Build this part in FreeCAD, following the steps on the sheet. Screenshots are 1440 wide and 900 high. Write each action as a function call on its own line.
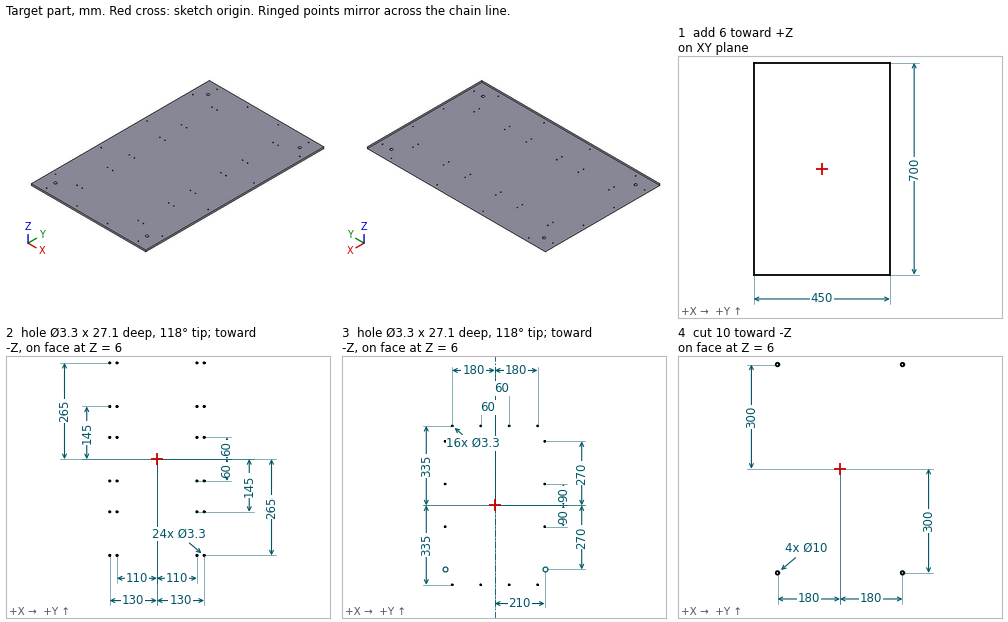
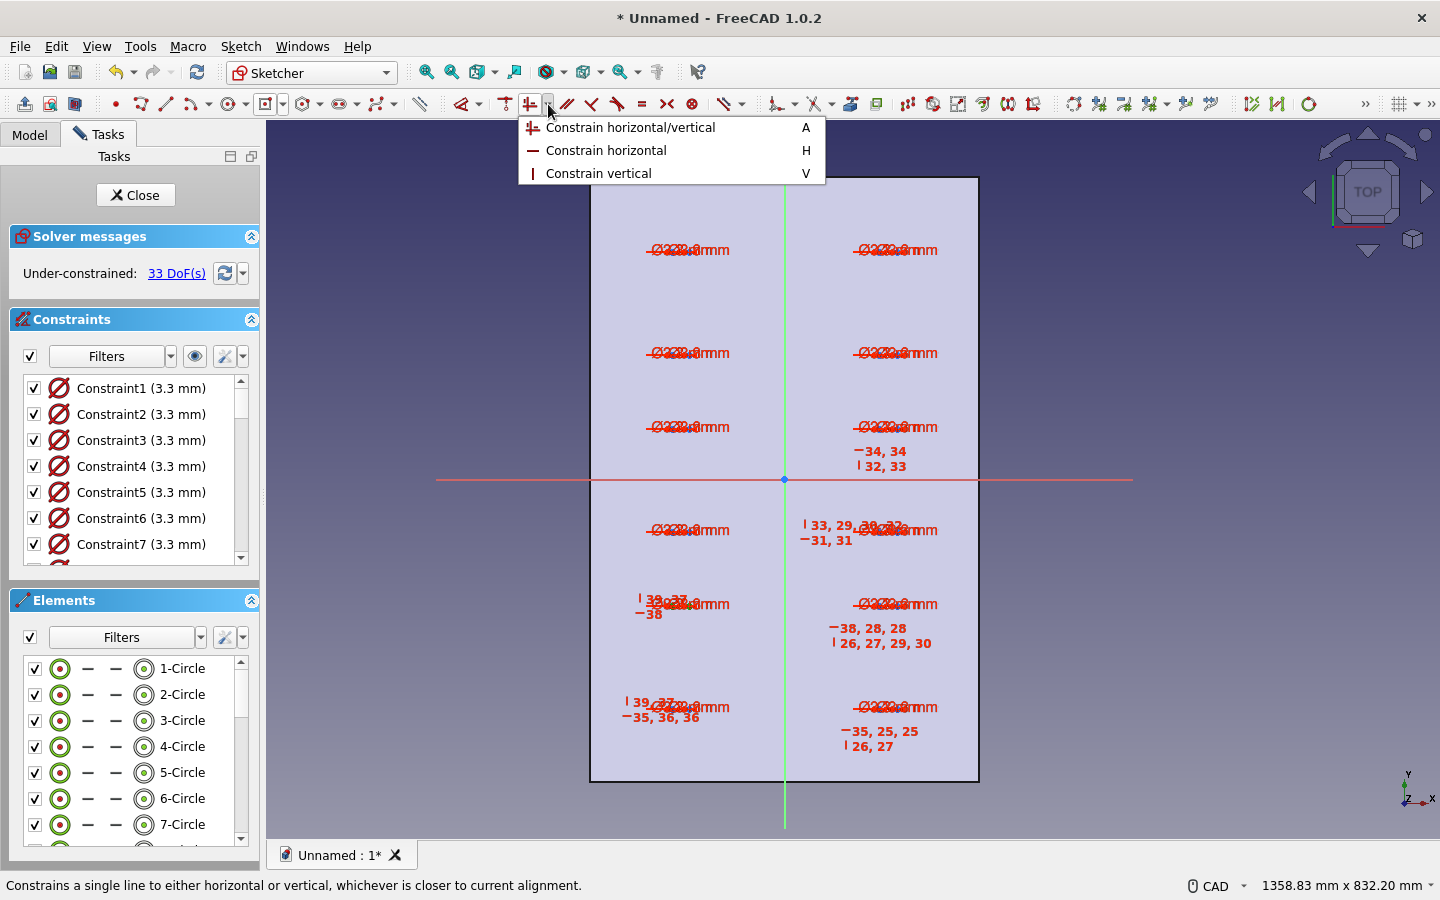
click(672, 150)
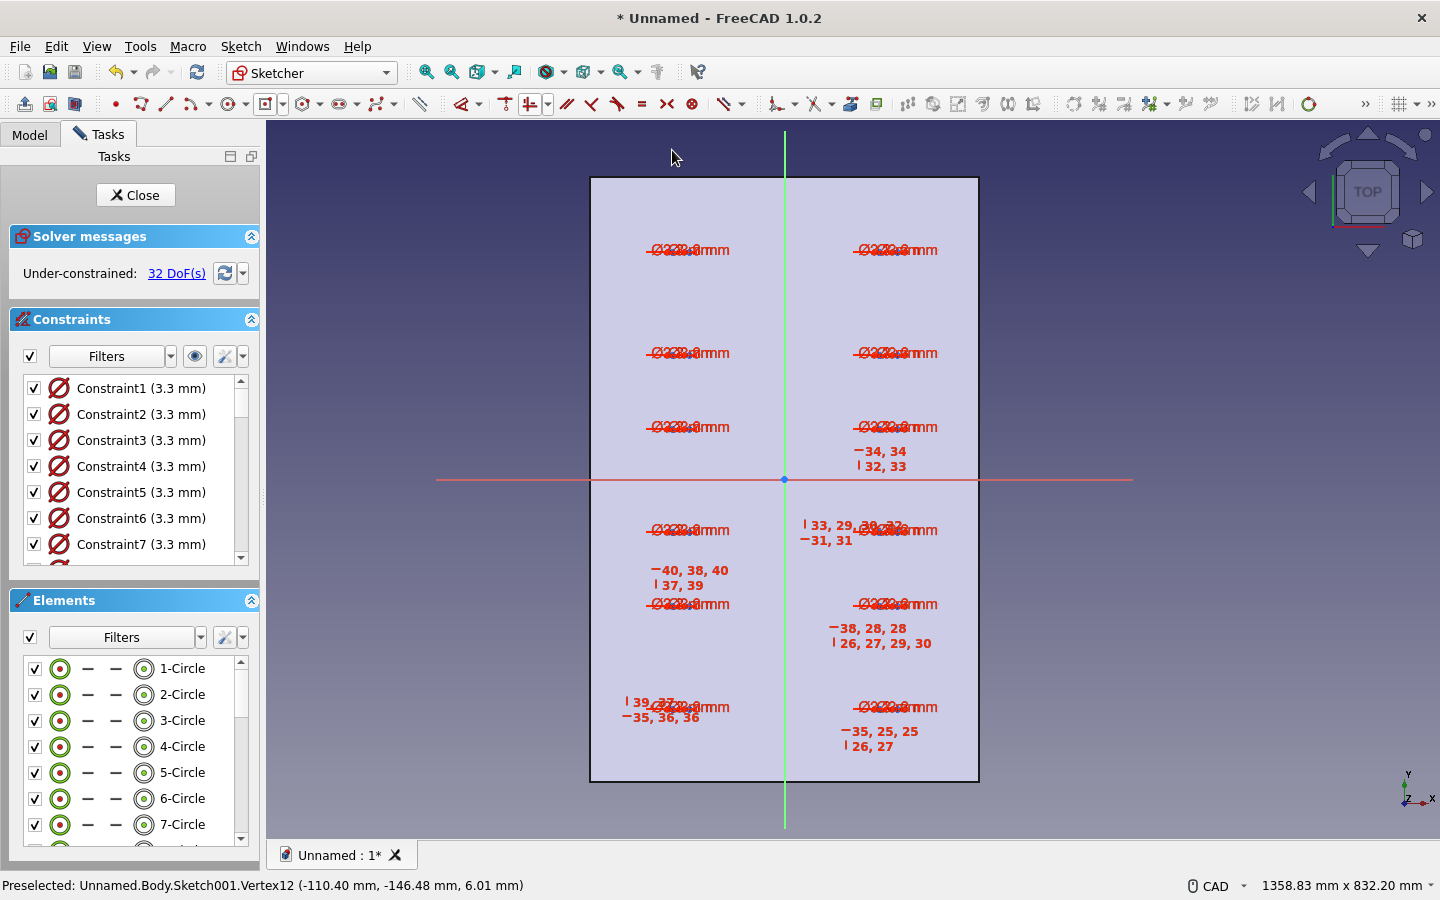
click(672, 606)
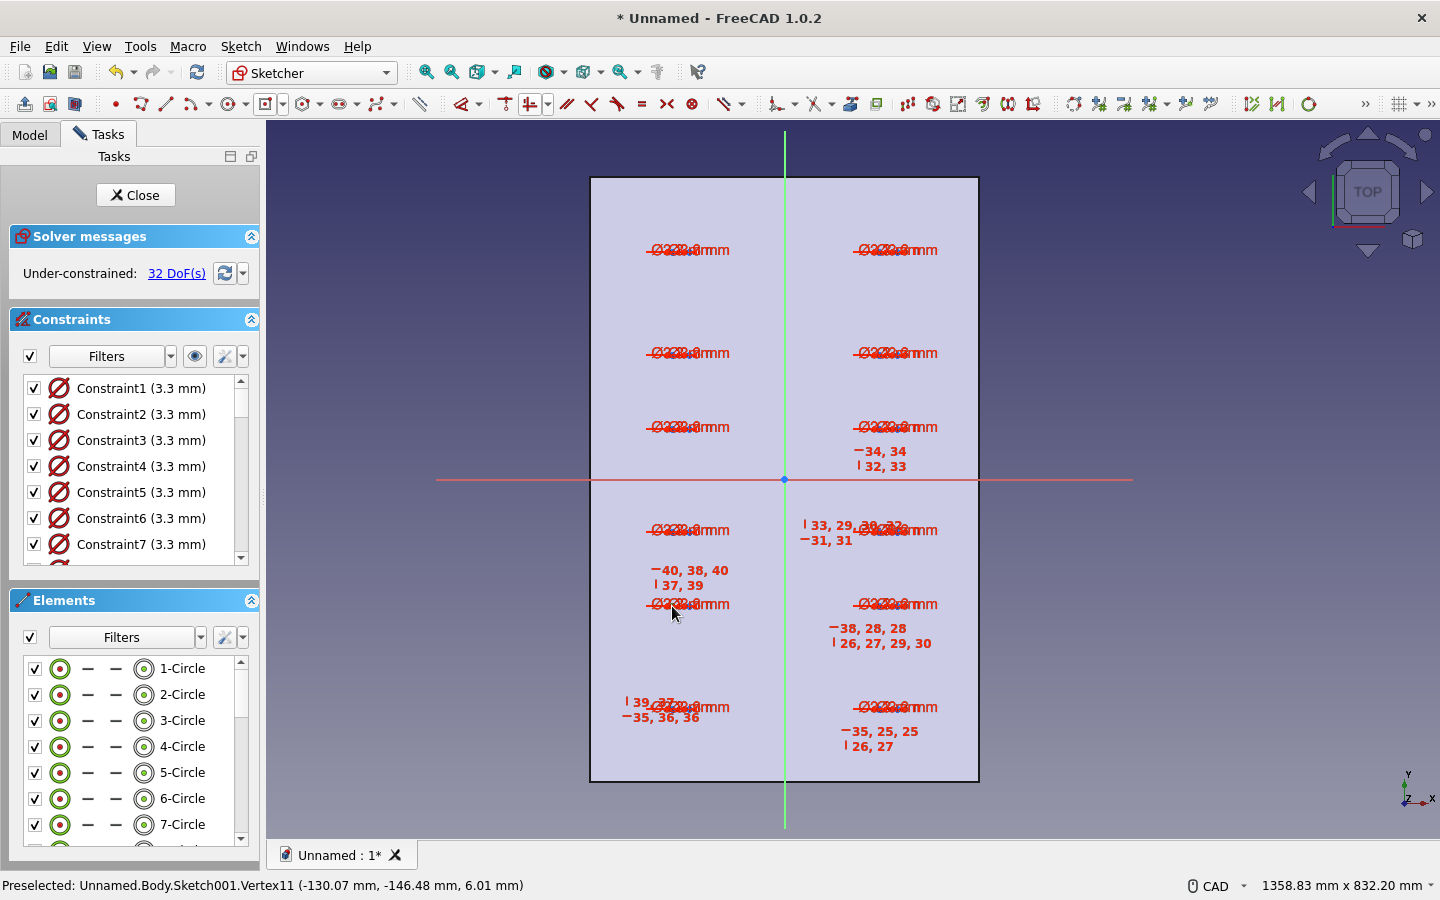
click(672, 532)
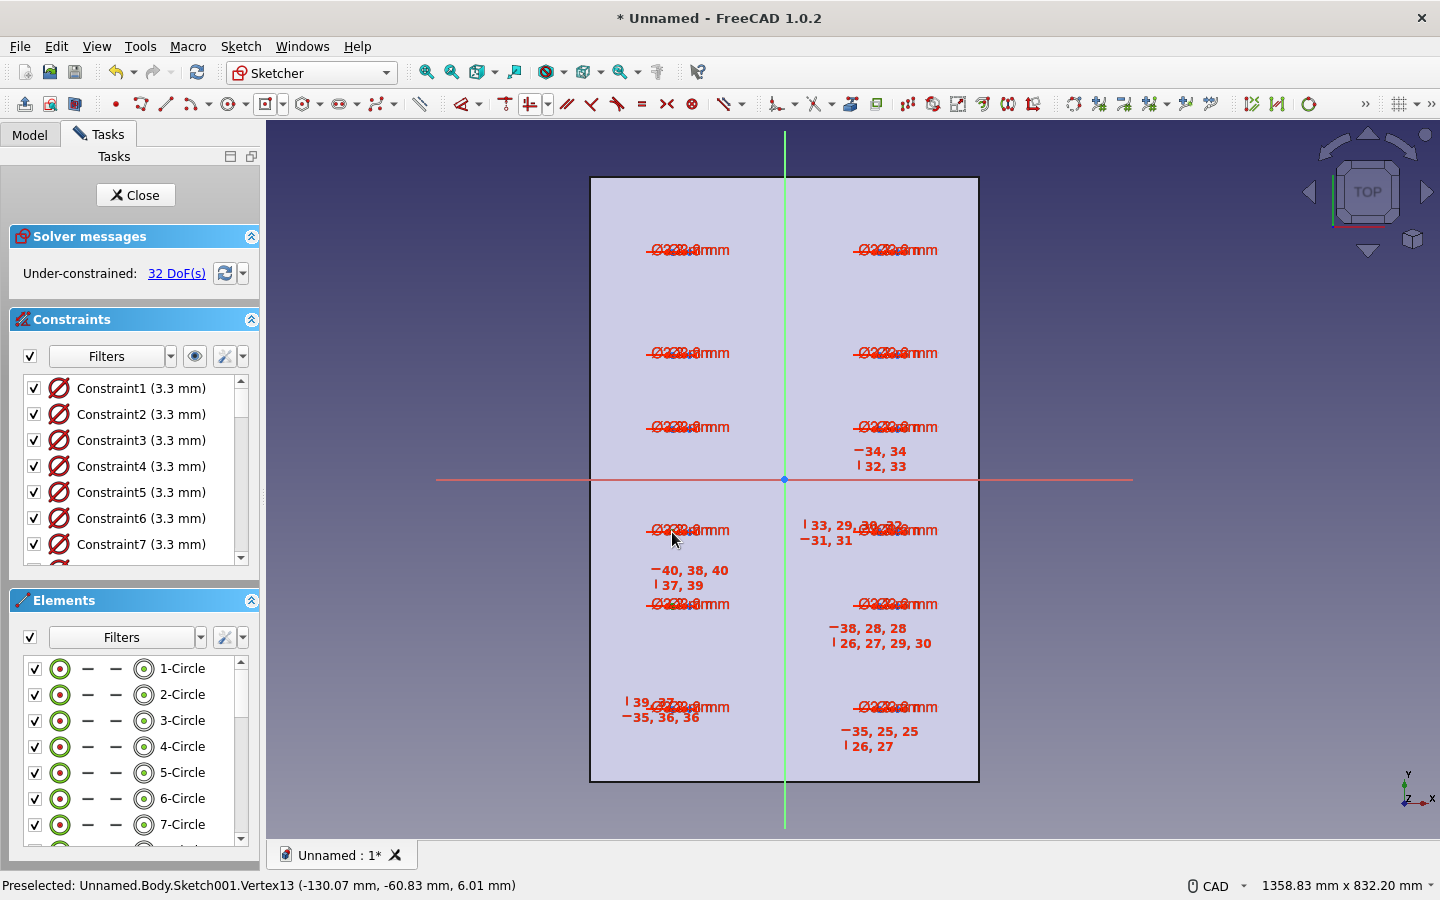
key(v)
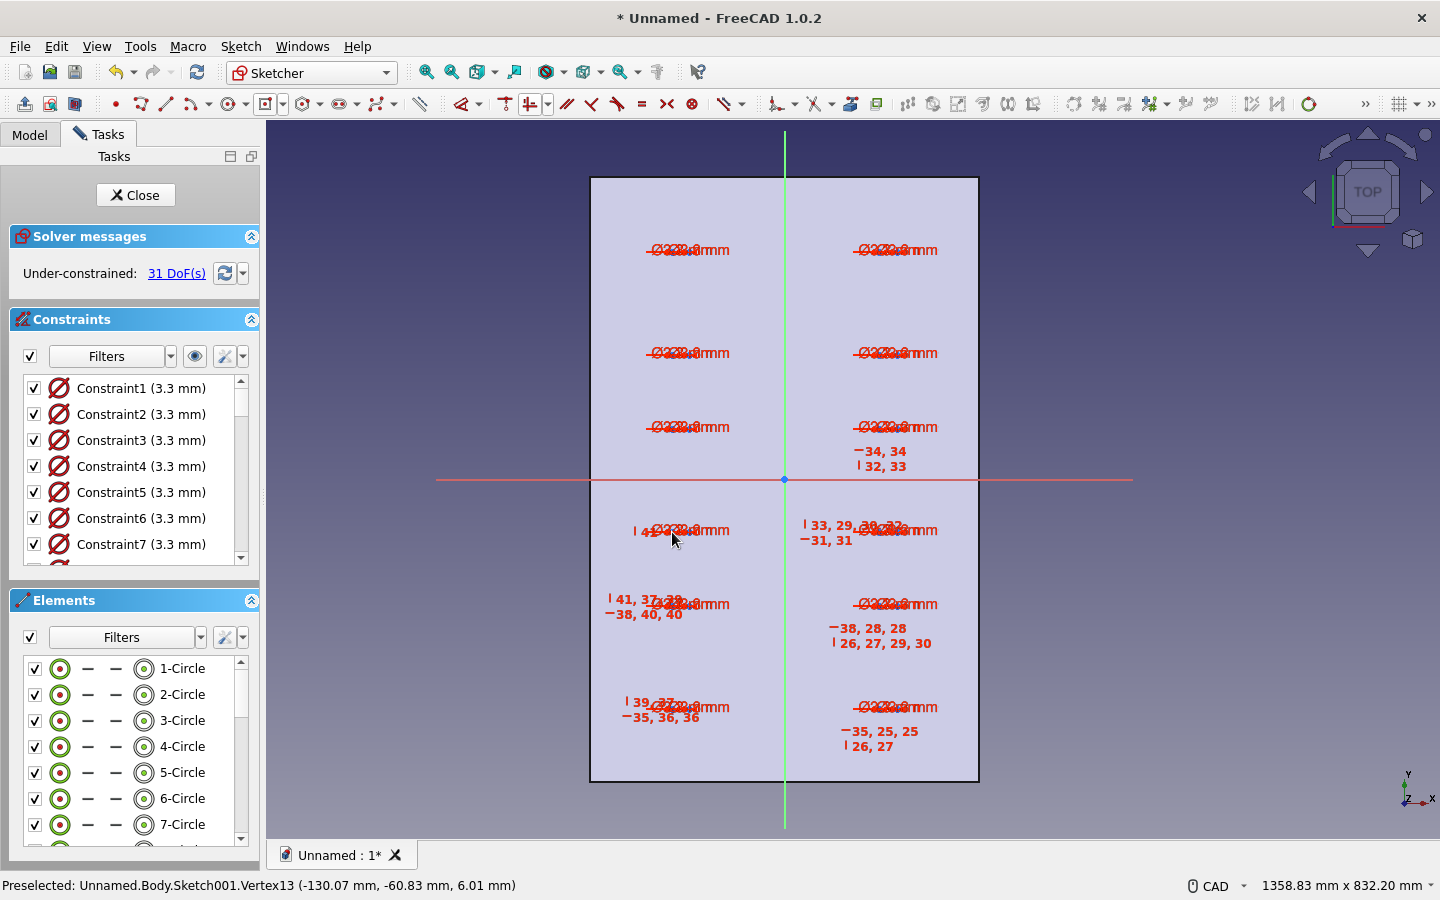
click(879, 532)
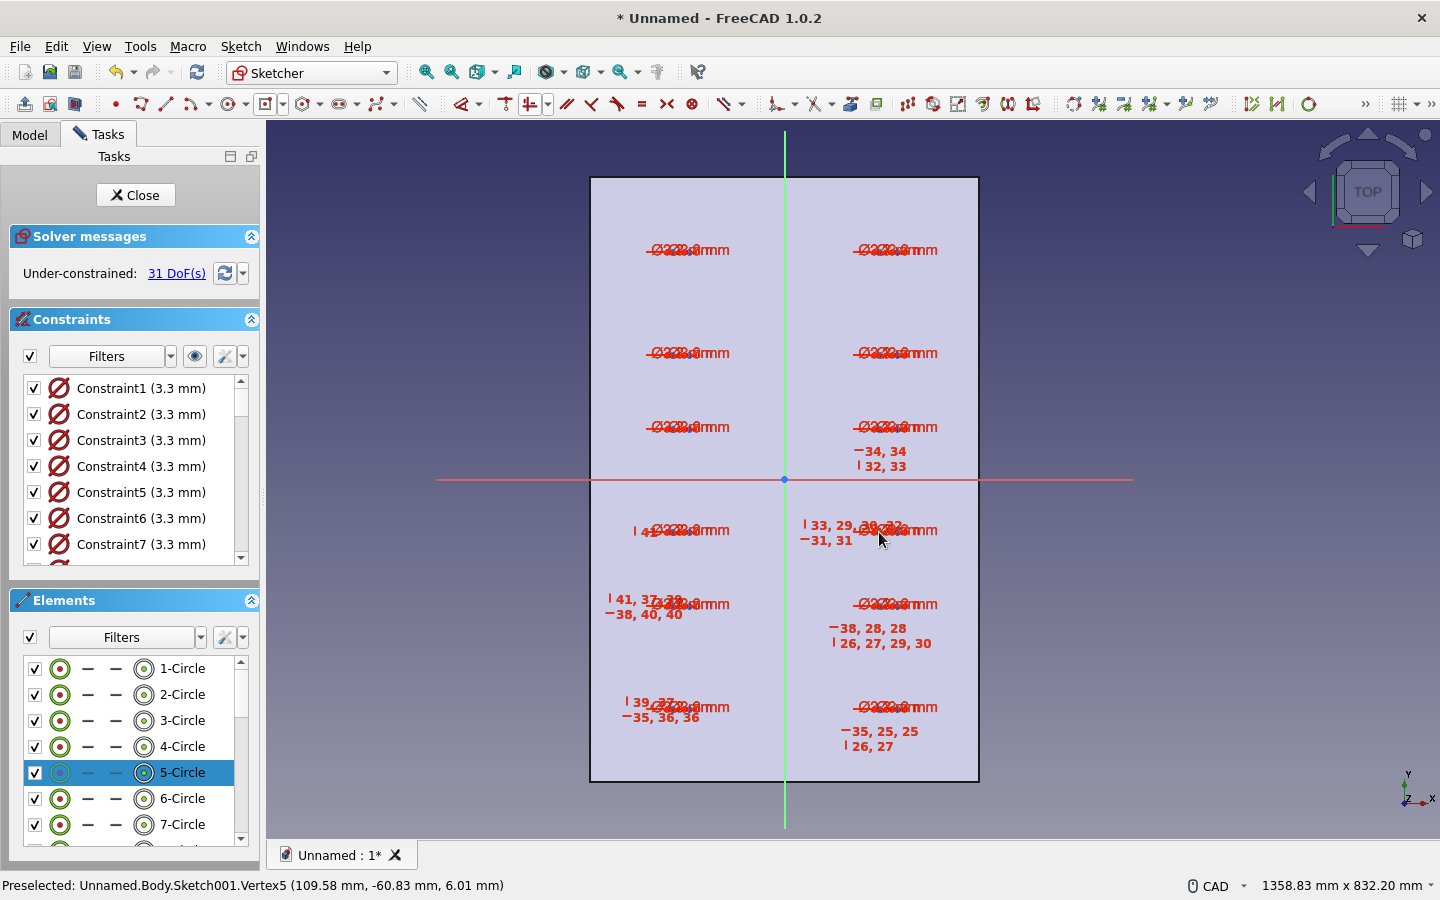
click(672, 532)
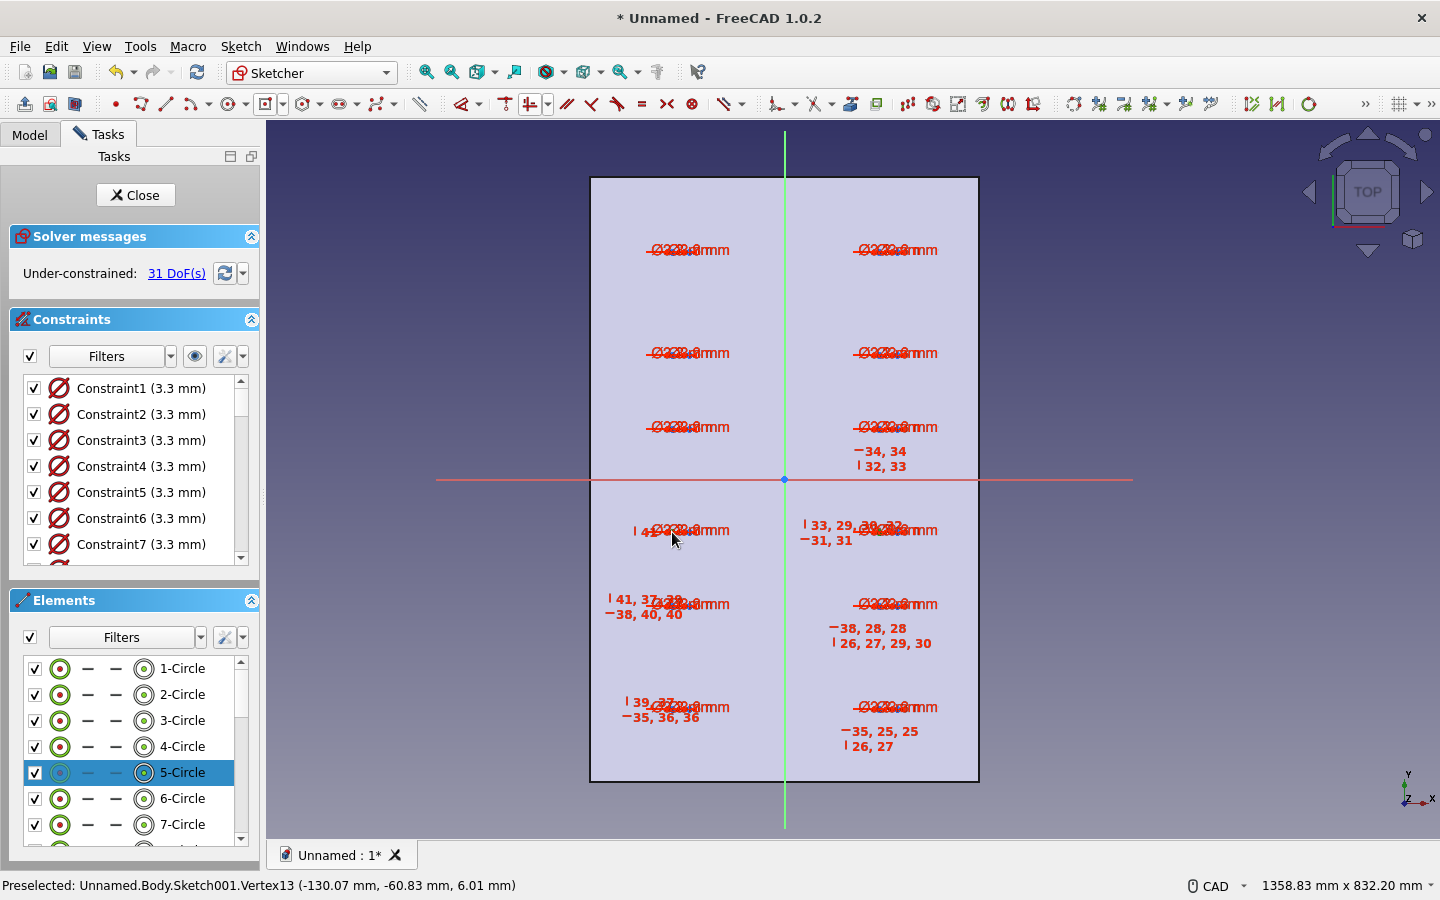
key(h)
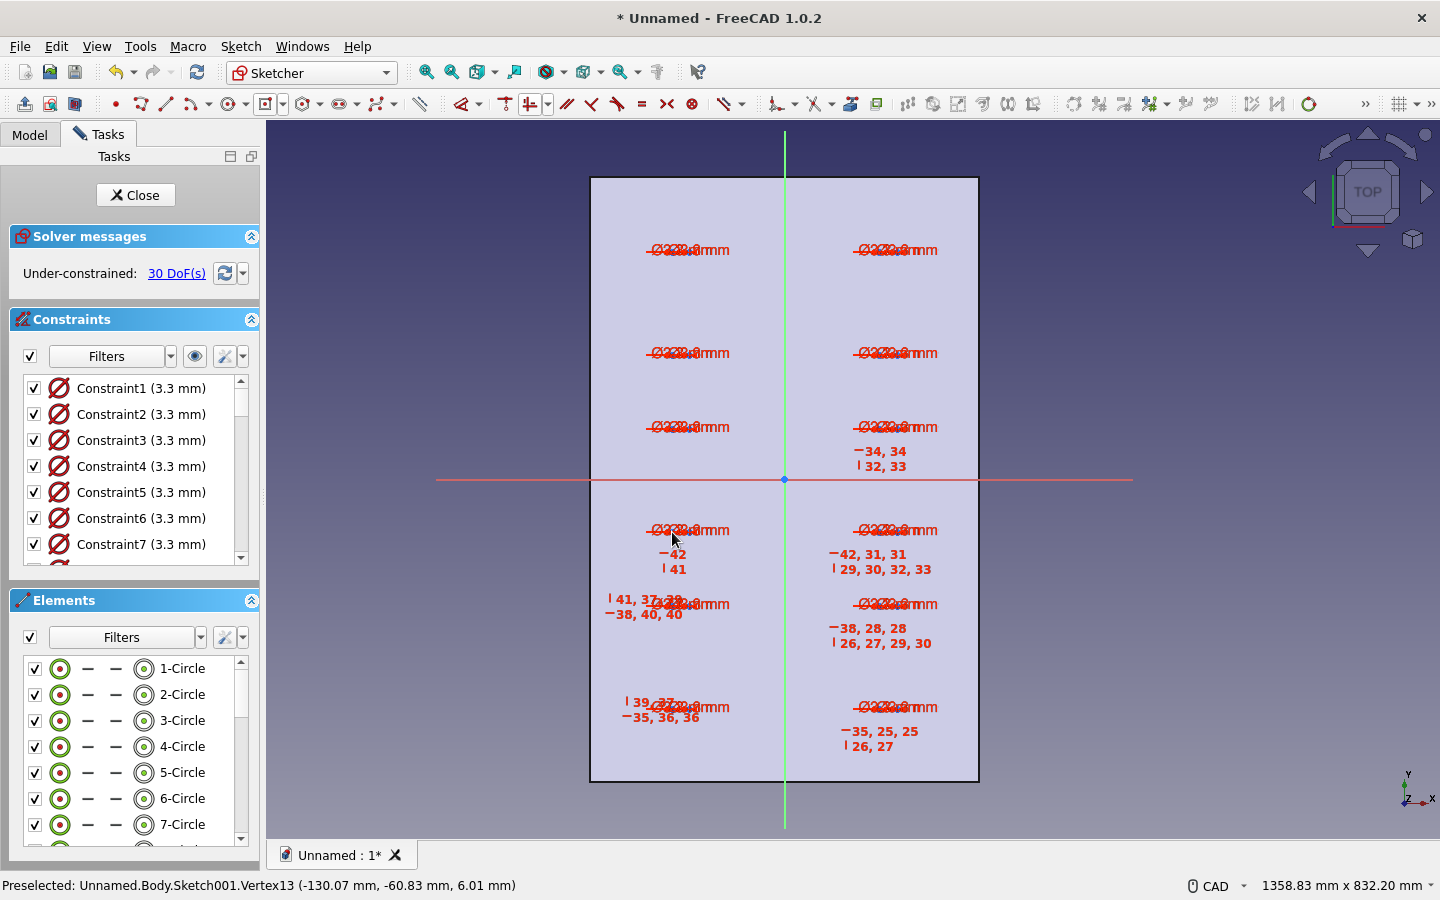
click(689, 606)